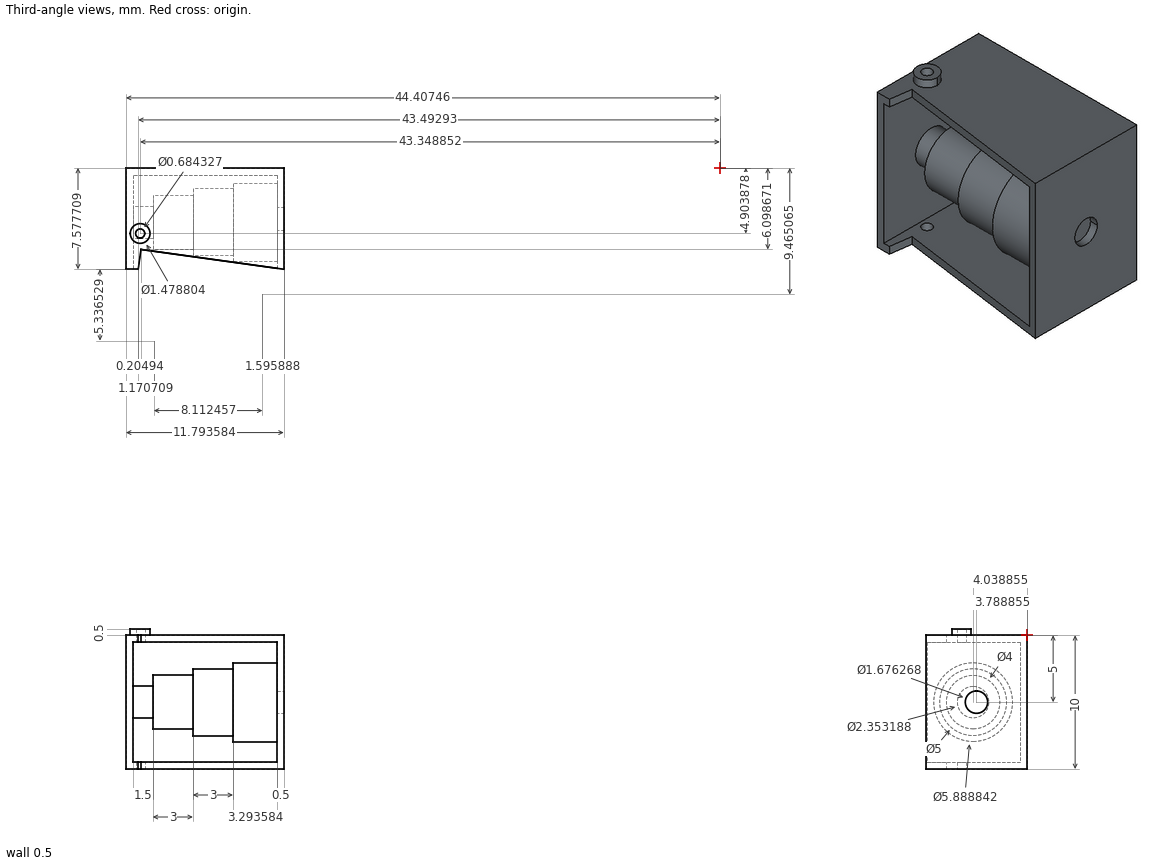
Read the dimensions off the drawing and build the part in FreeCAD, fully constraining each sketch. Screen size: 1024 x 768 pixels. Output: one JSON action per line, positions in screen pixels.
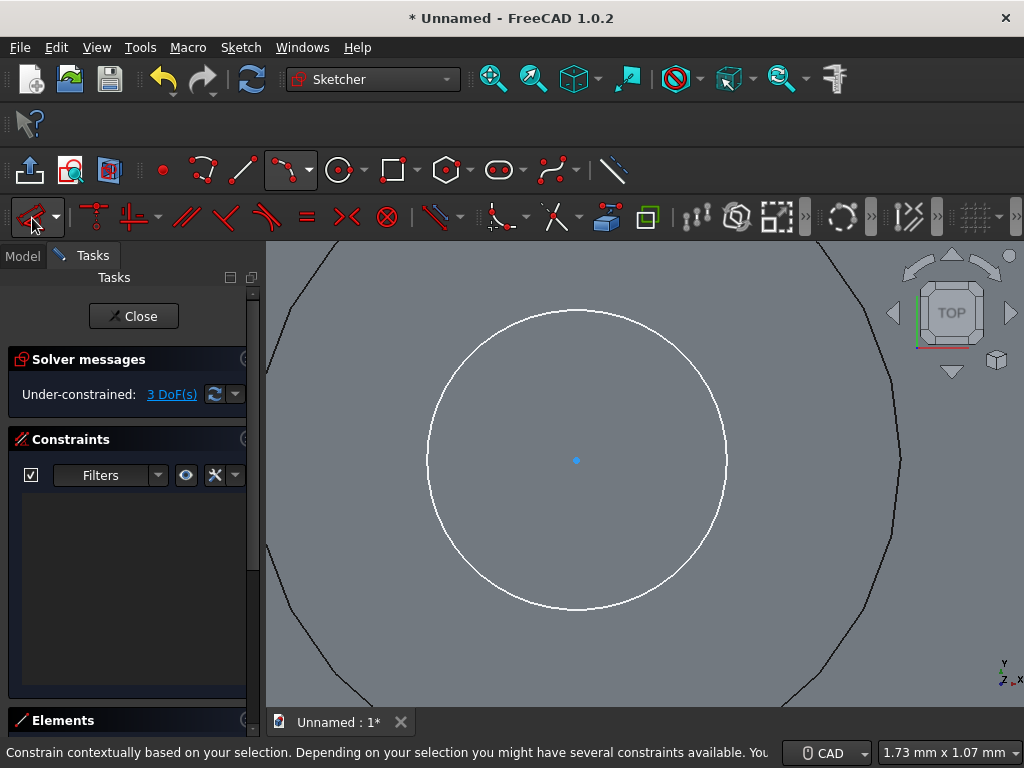
{"action": "left_click", "coordinate": [683, 354]}
{"action": "left_click", "coordinate": [706, 331]}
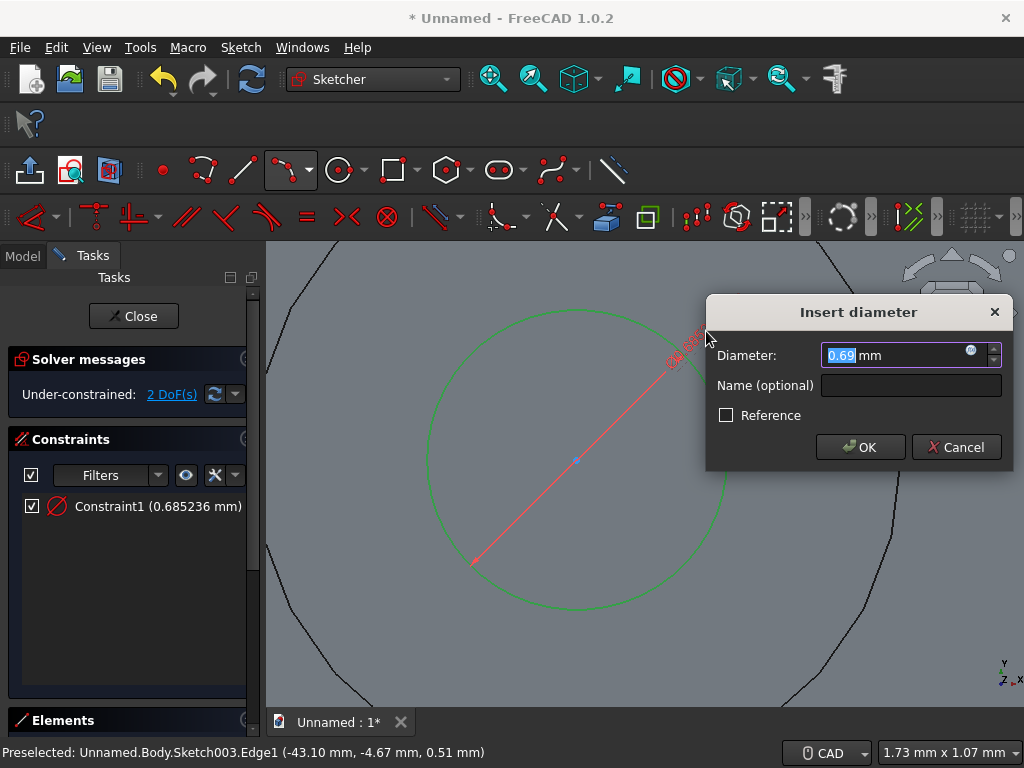
{"action": "type", "text": "0.684327"}
{"action": "key", "text": "Return"}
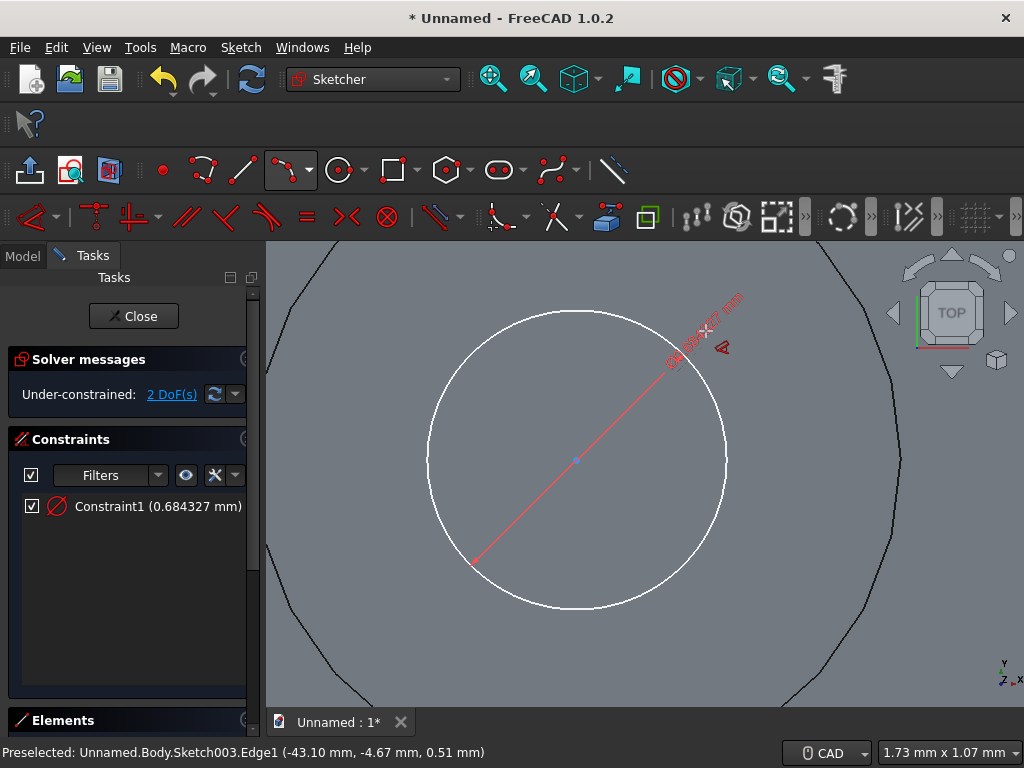
{"action": "left_click", "coordinate": [577, 460]}
{"action": "left_click", "coordinate": [543, 365]}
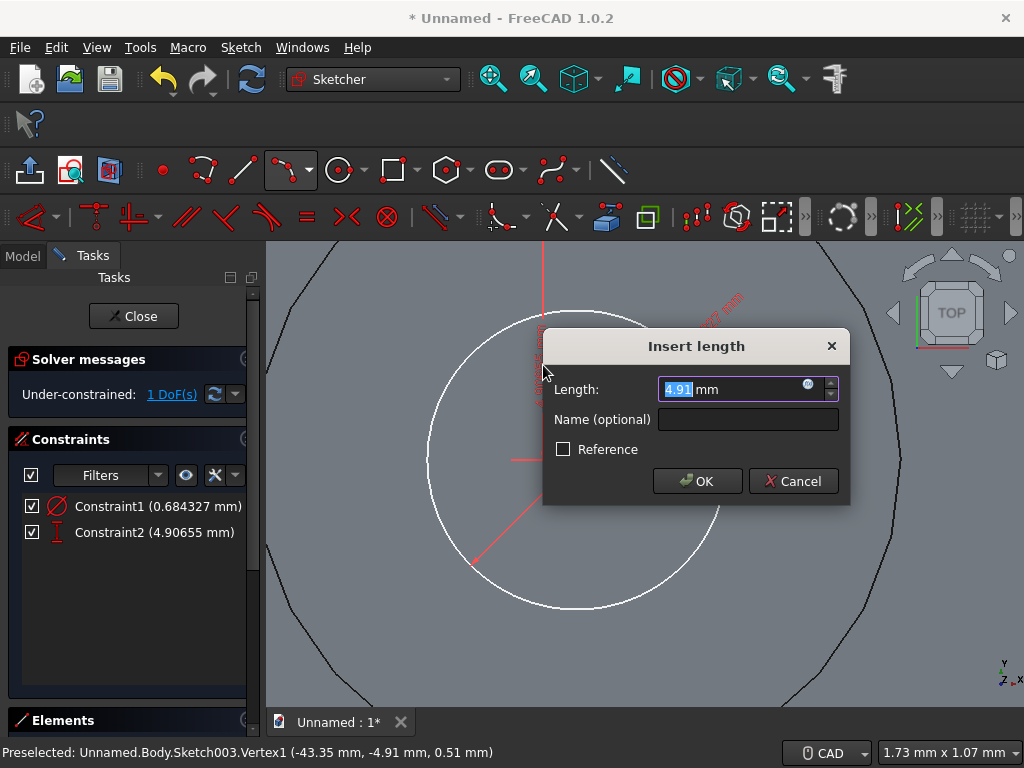
{"action": "type", "text": "4.903878"}
{"action": "key", "text": "Return"}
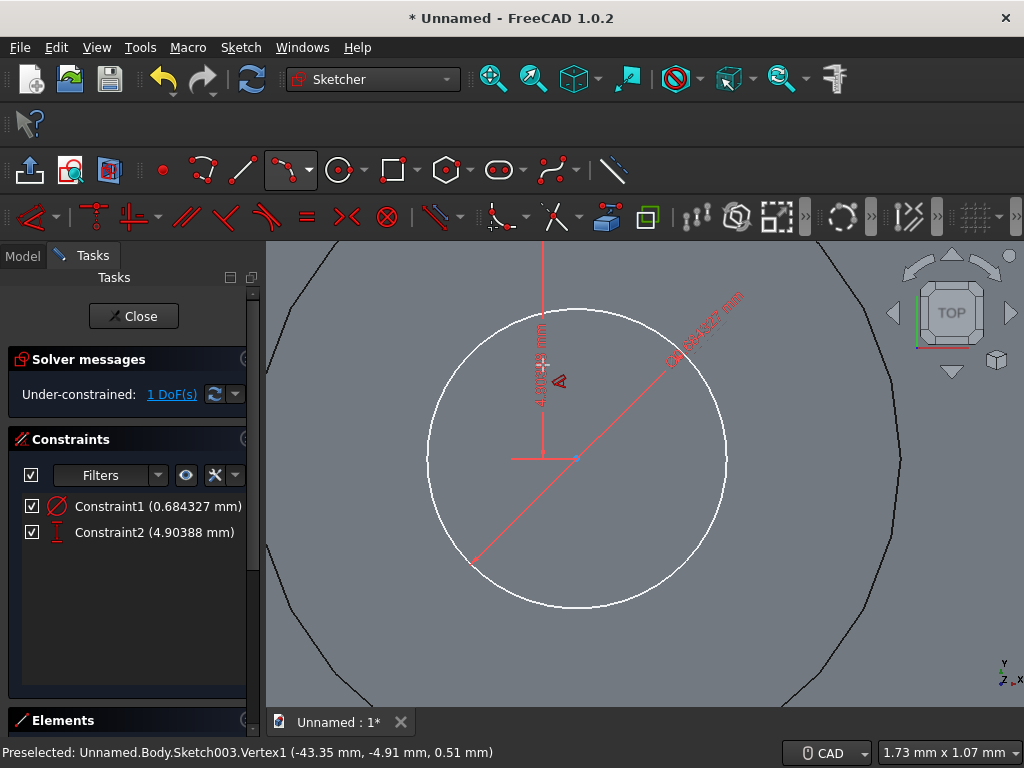
{"action": "left_click", "coordinate": [577, 459]}
{"action": "left_click", "coordinate": [653, 493]}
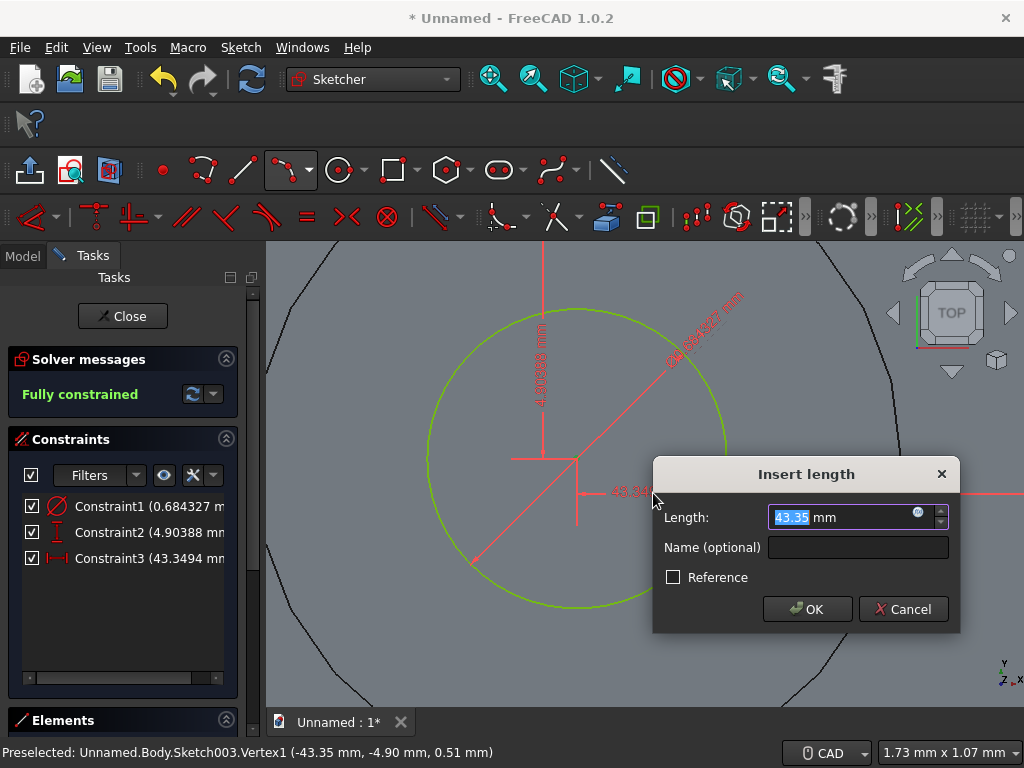
{"action": "type", "text": "43.348852"}
{"action": "key", "text": "Return"}
{"action": "key", "text": "Escape"}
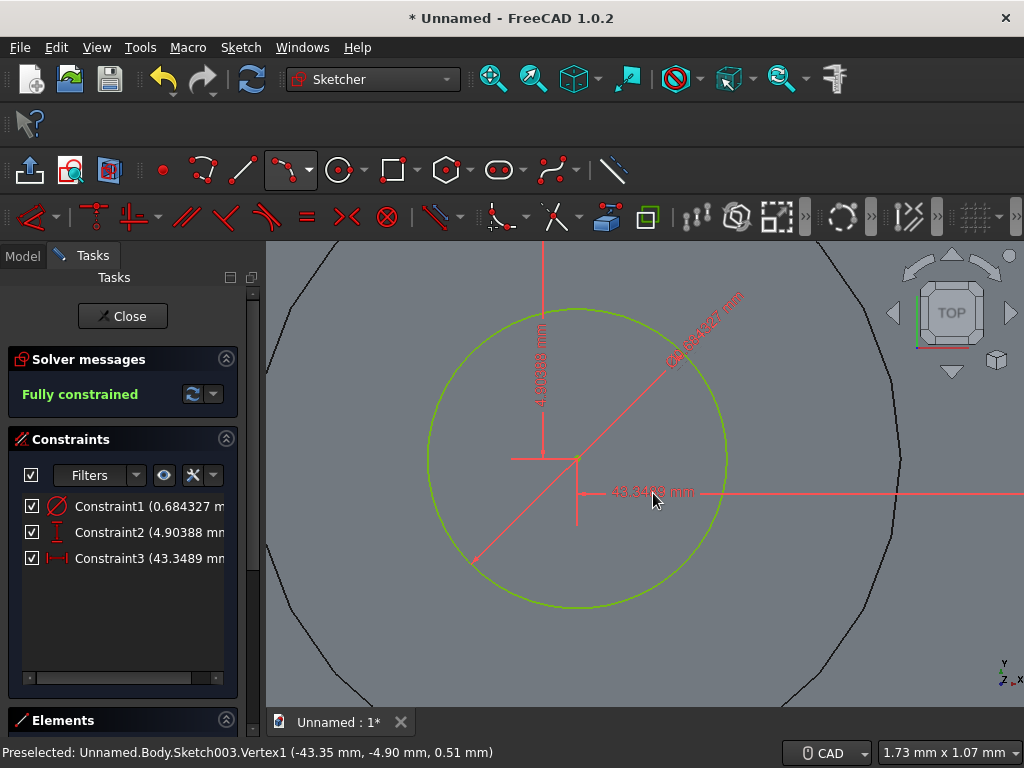
{"action": "left_click", "coordinate": [123, 316]}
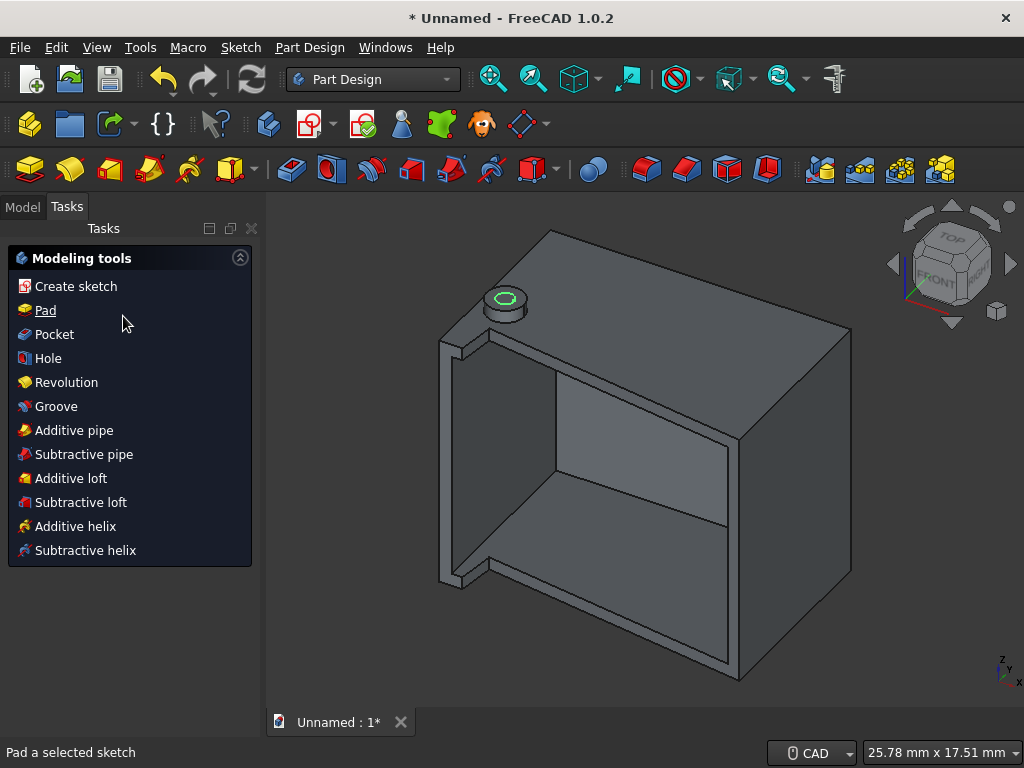
{"action": "left_click", "coordinate": [292, 170]}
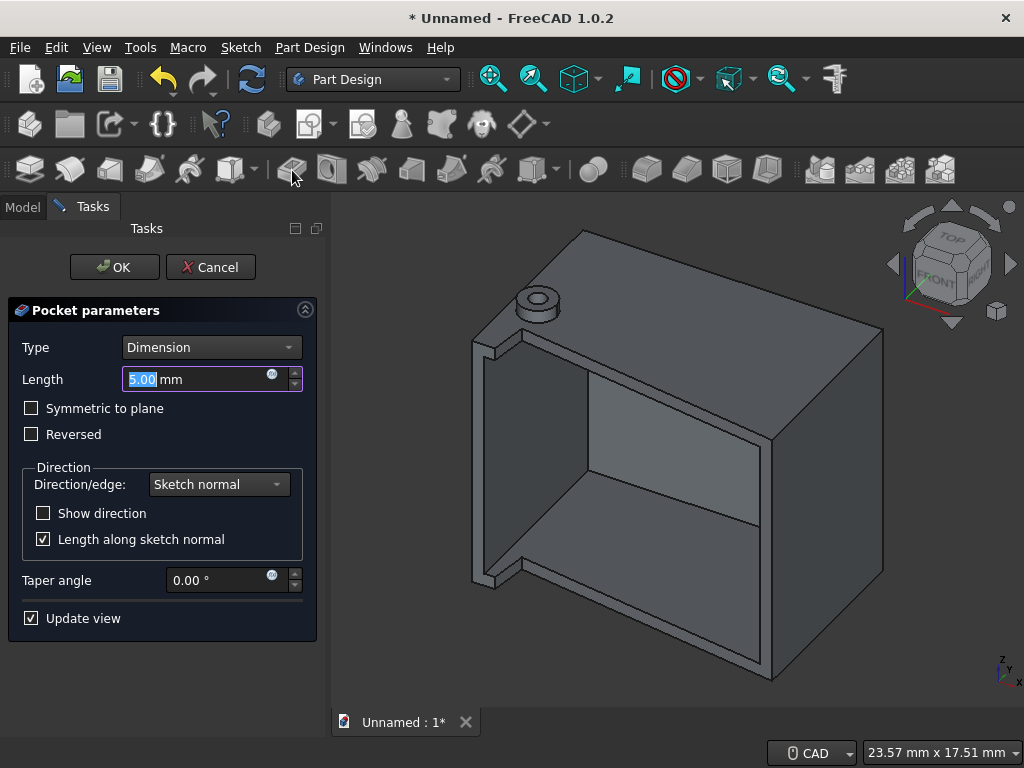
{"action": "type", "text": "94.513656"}
{"action": "key", "text": "Tab"}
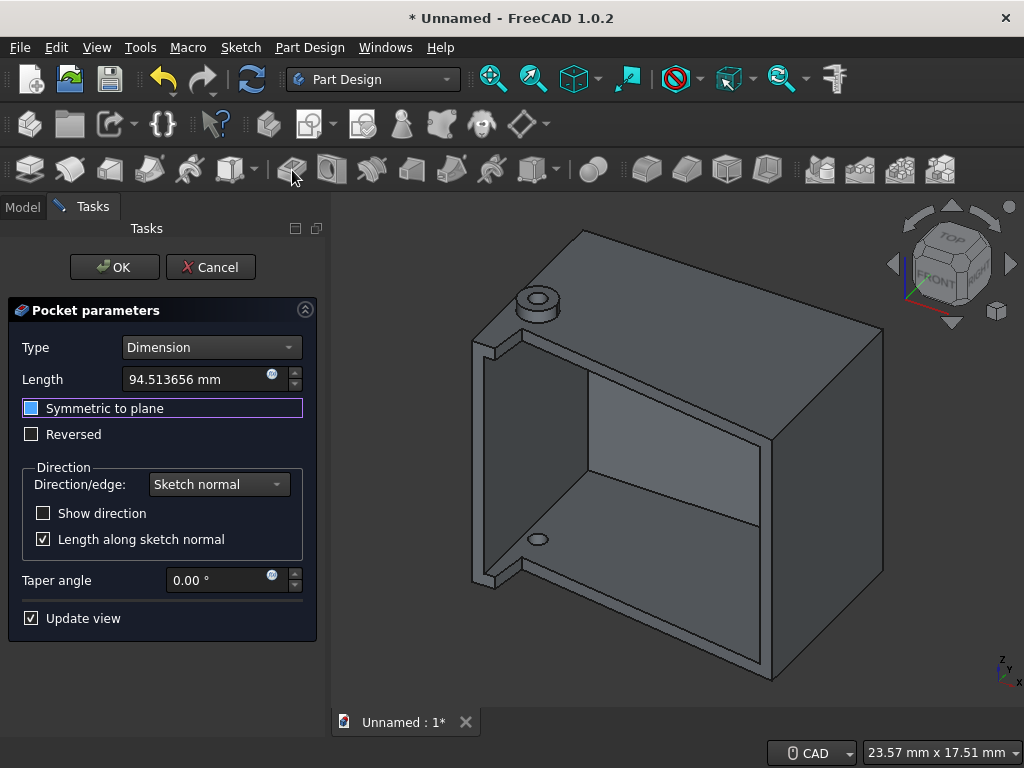
{"action": "left_click", "coordinate": [30, 408]}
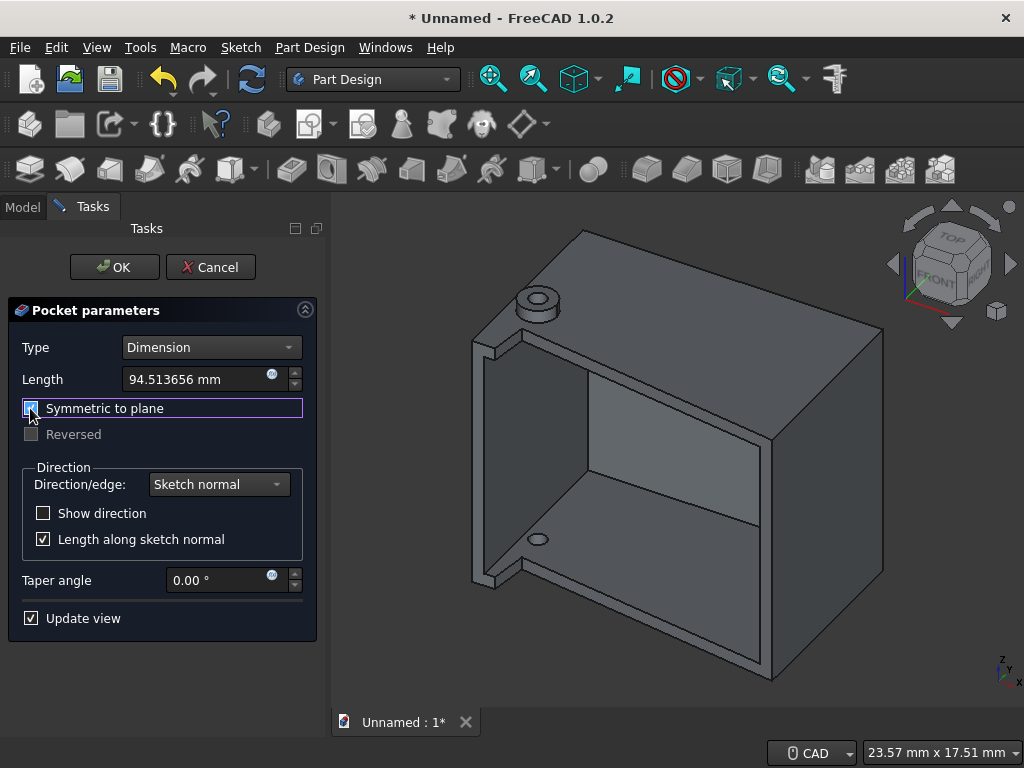
{"action": "left_click", "coordinate": [115, 267]}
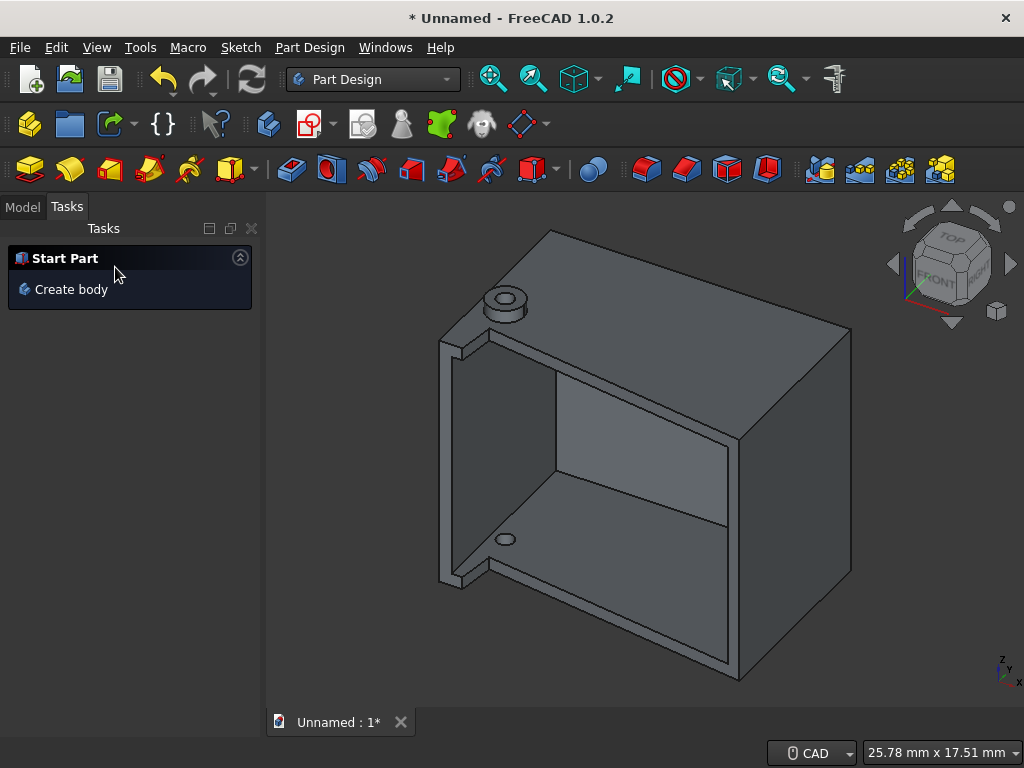
{"action": "left_click", "coordinate": [795, 504]}